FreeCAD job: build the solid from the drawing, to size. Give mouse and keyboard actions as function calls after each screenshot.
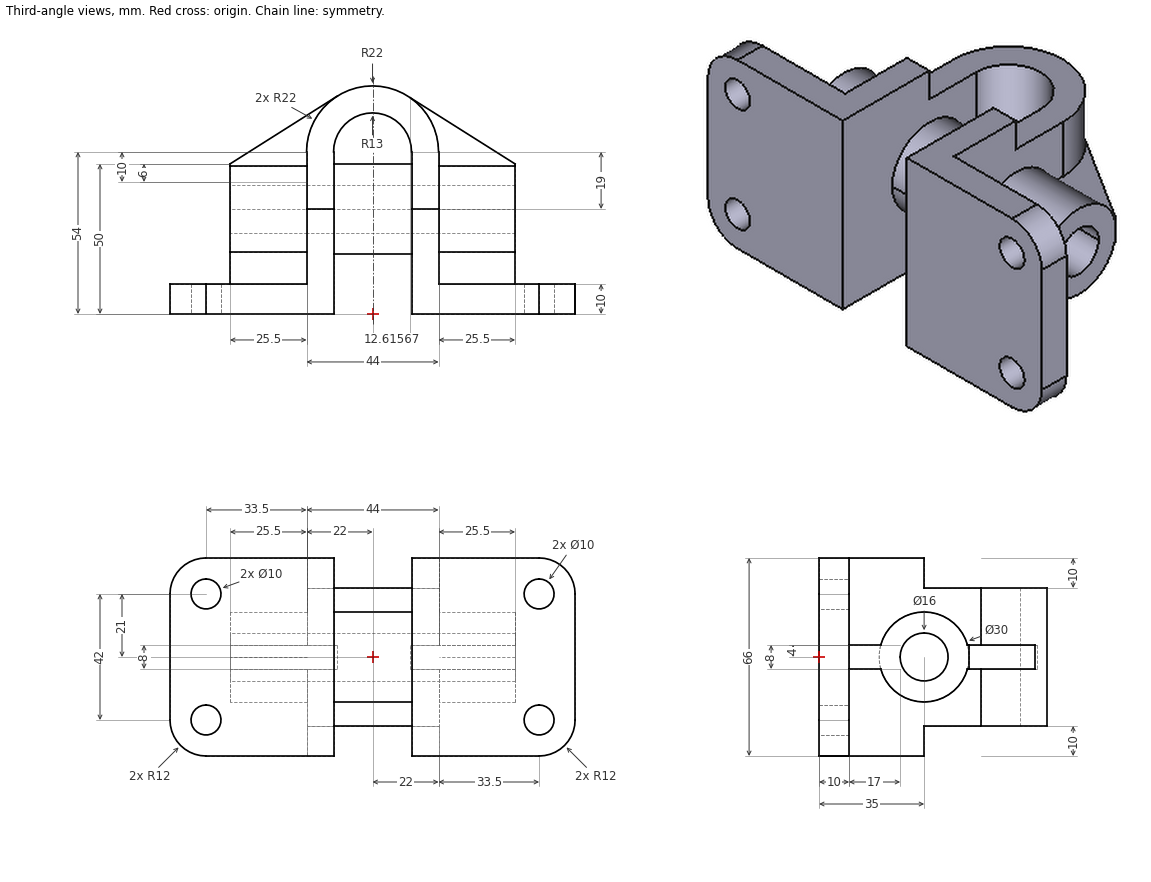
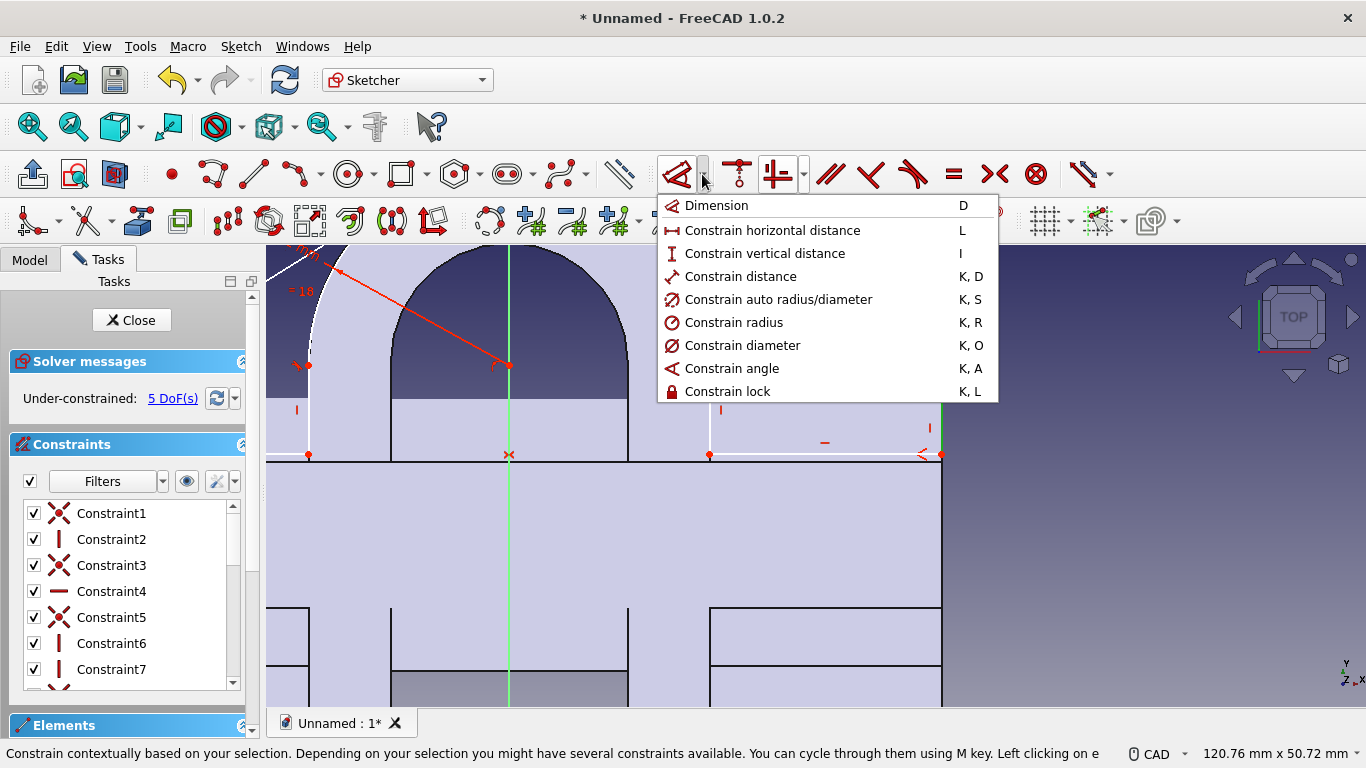
click(828, 254)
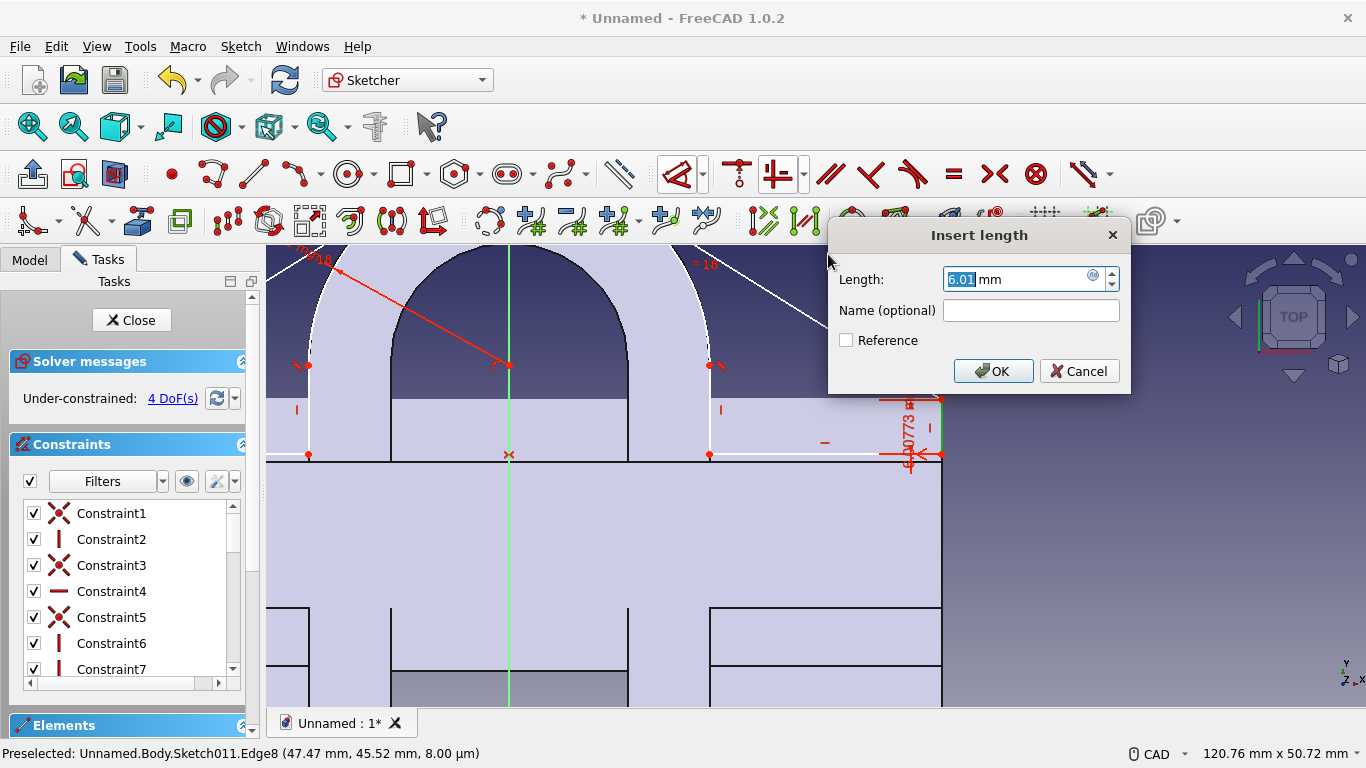
text(6)
key(Return)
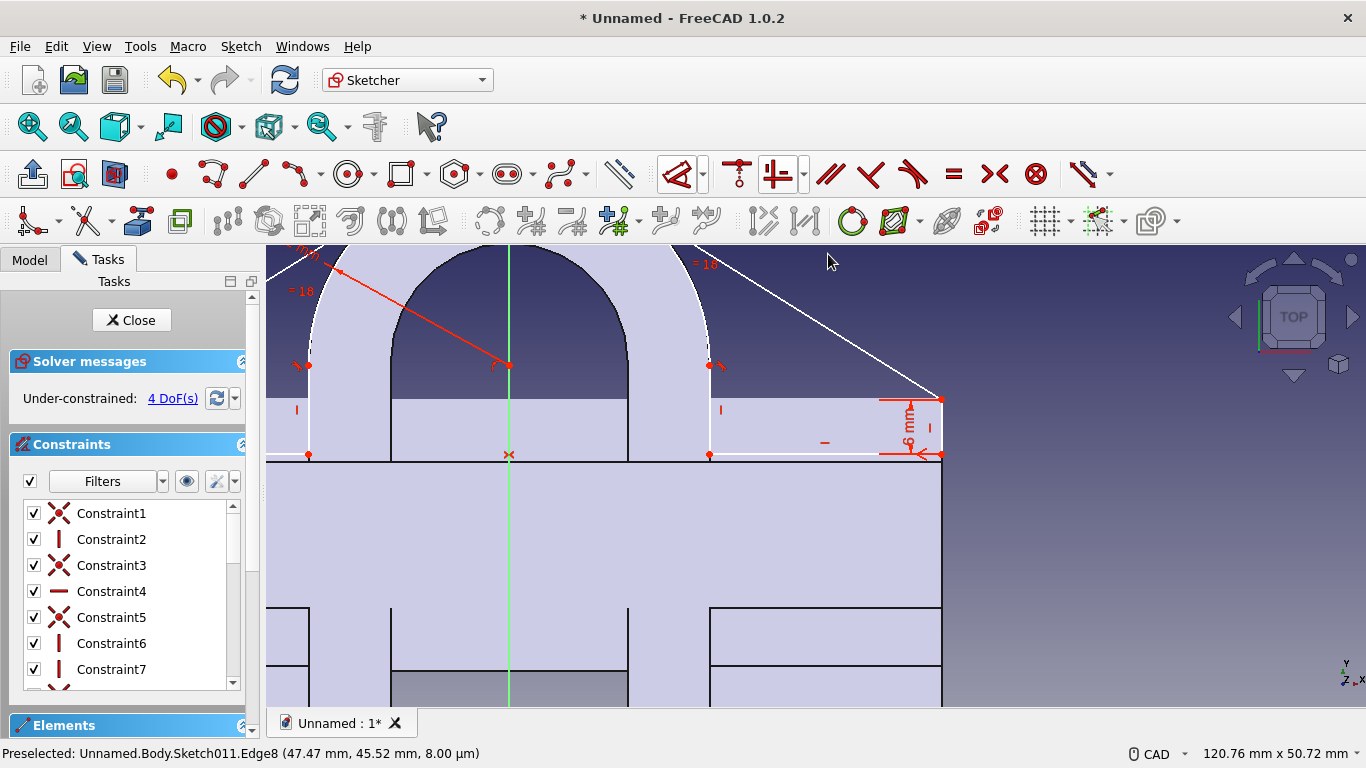
click(309, 428)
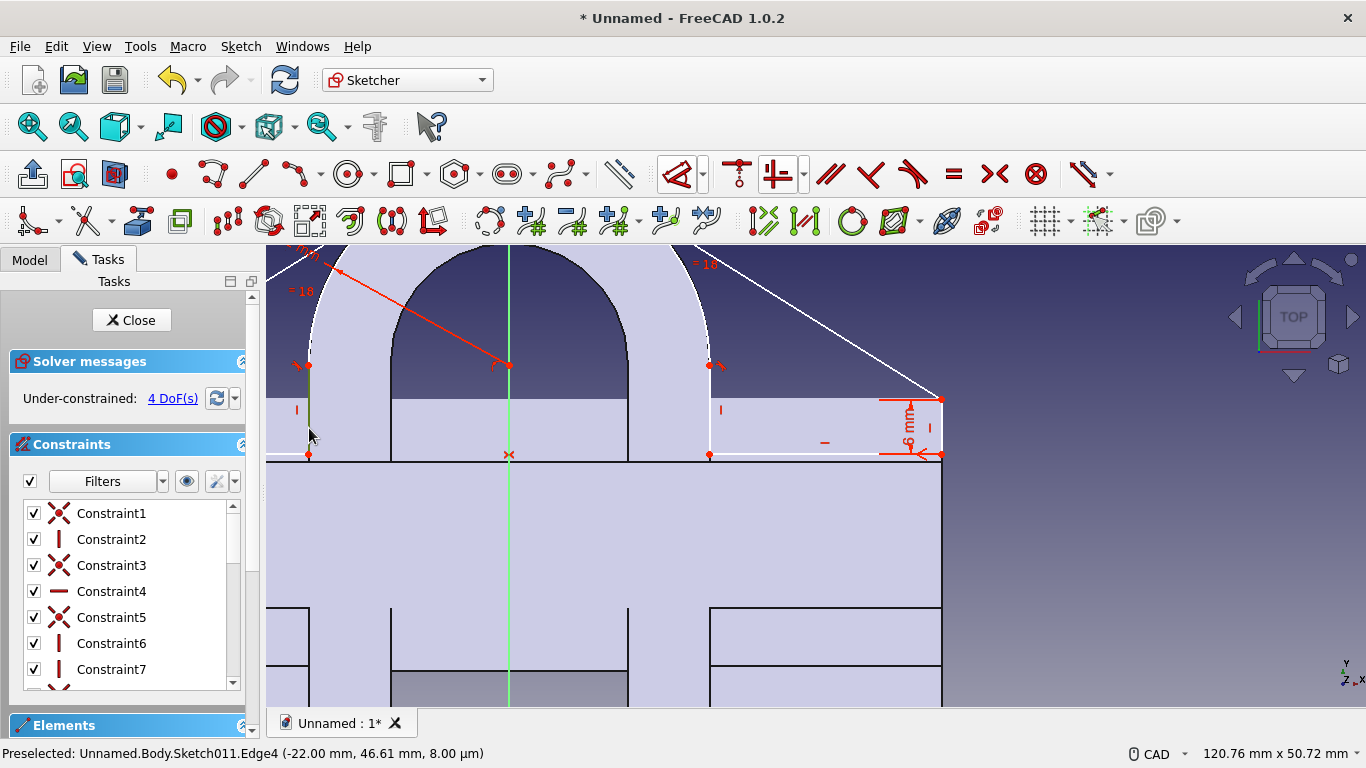
click(702, 174)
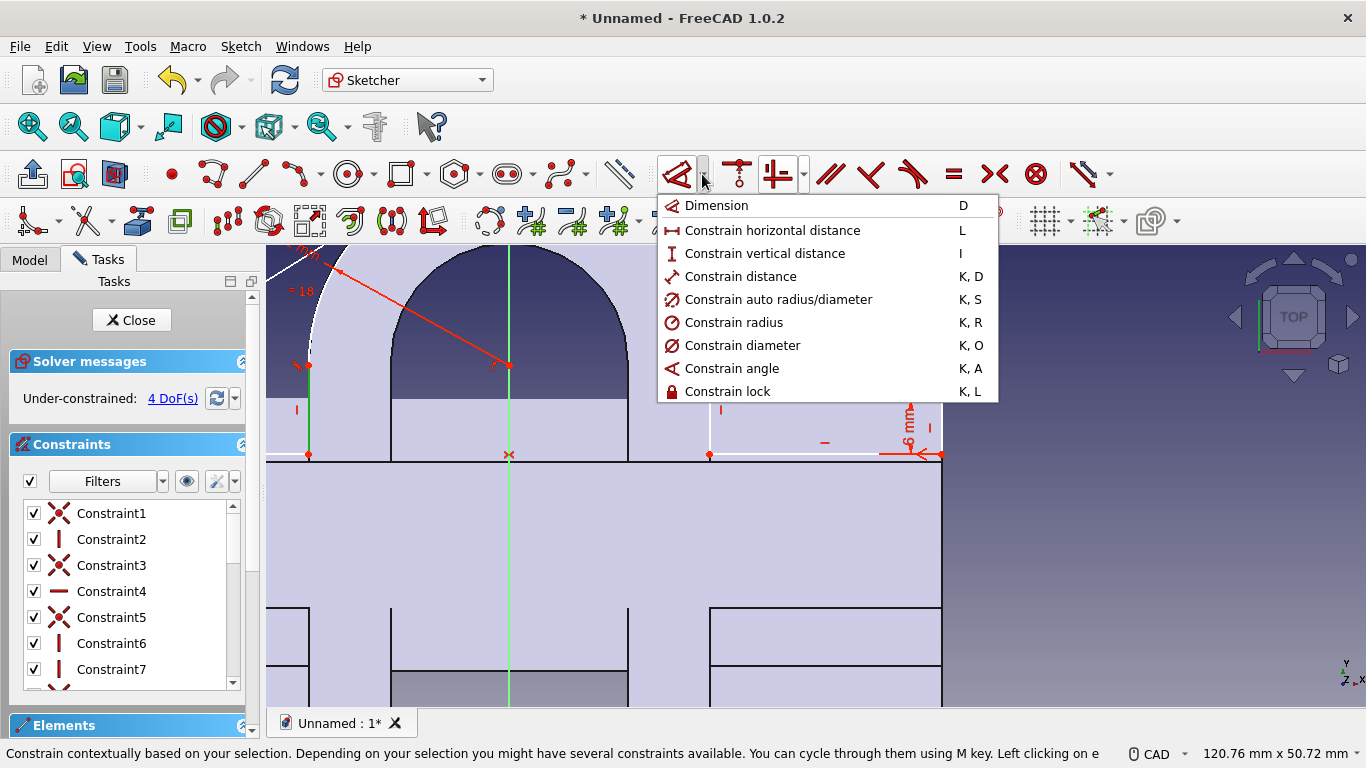
click(828, 254)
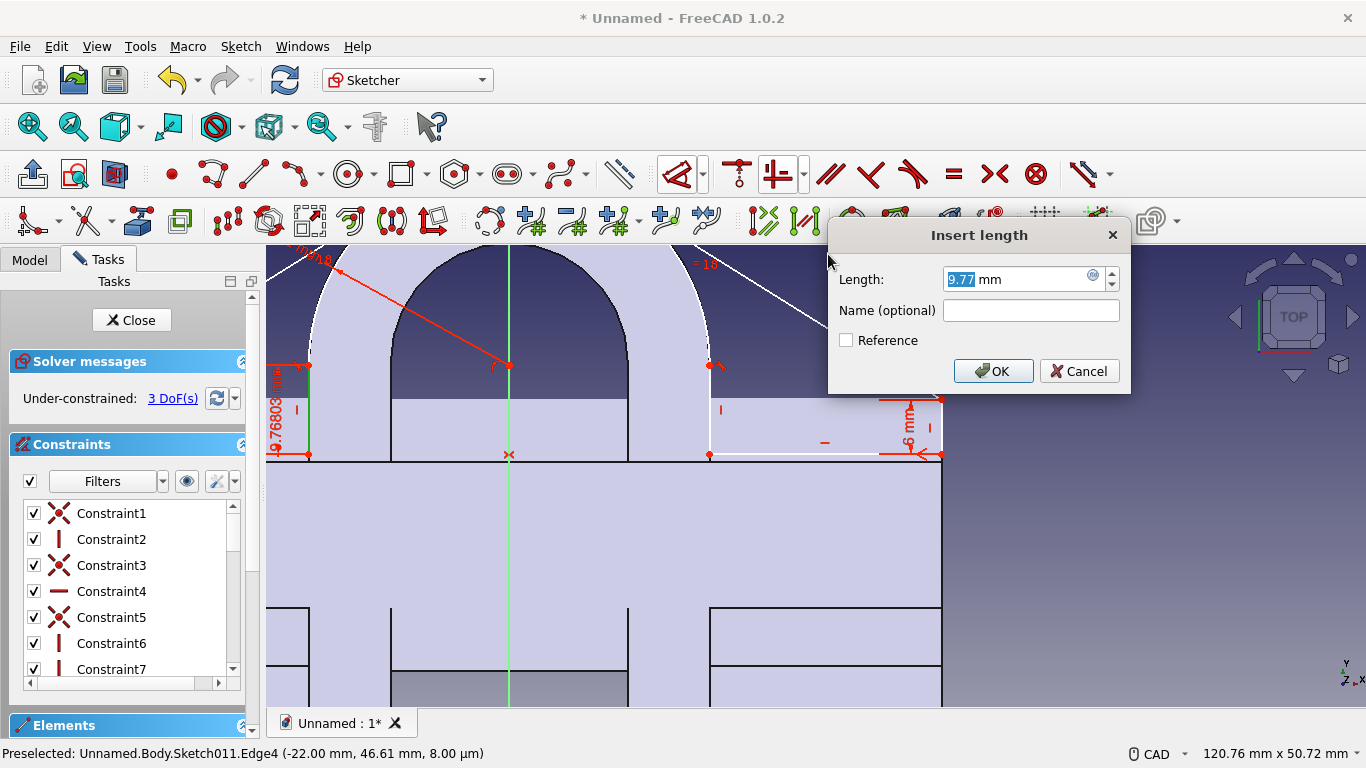
text(10)
key(Return)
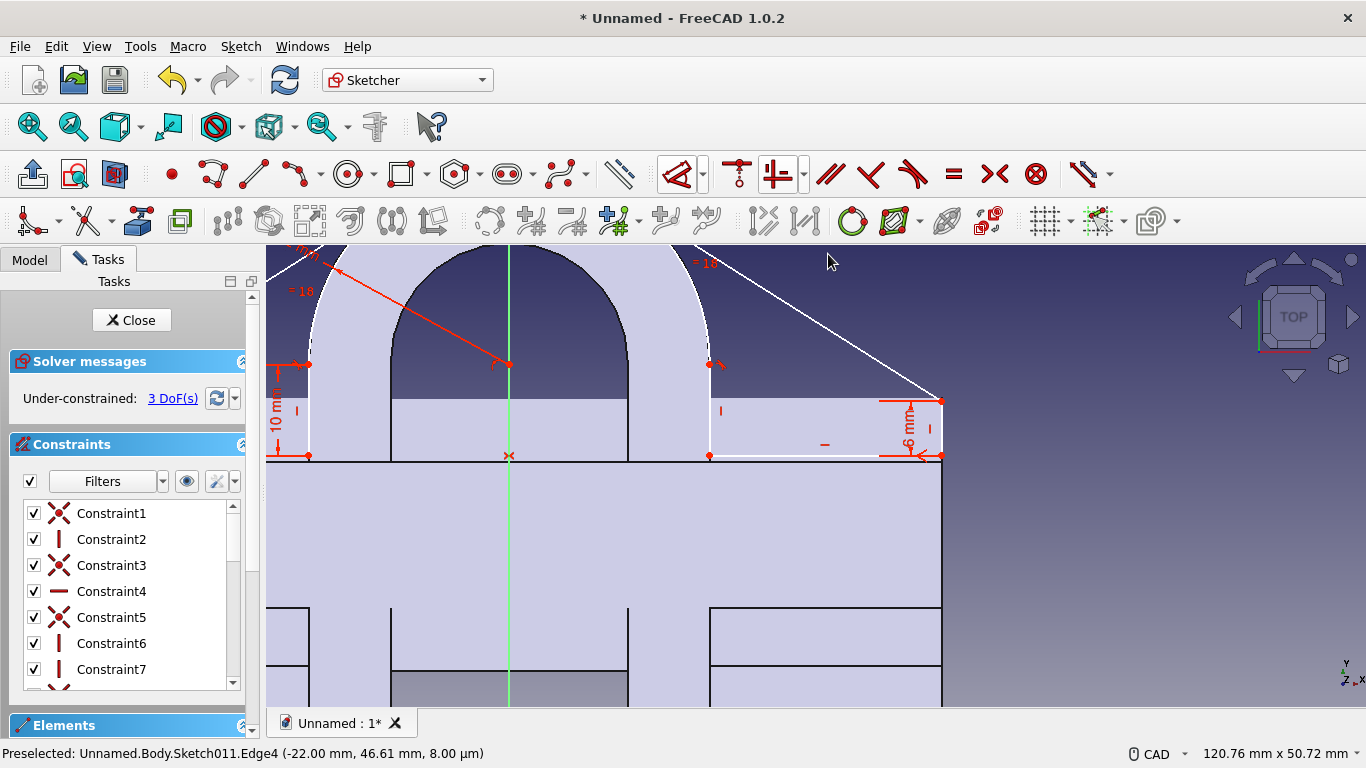
scroll(942, 438, down, 4)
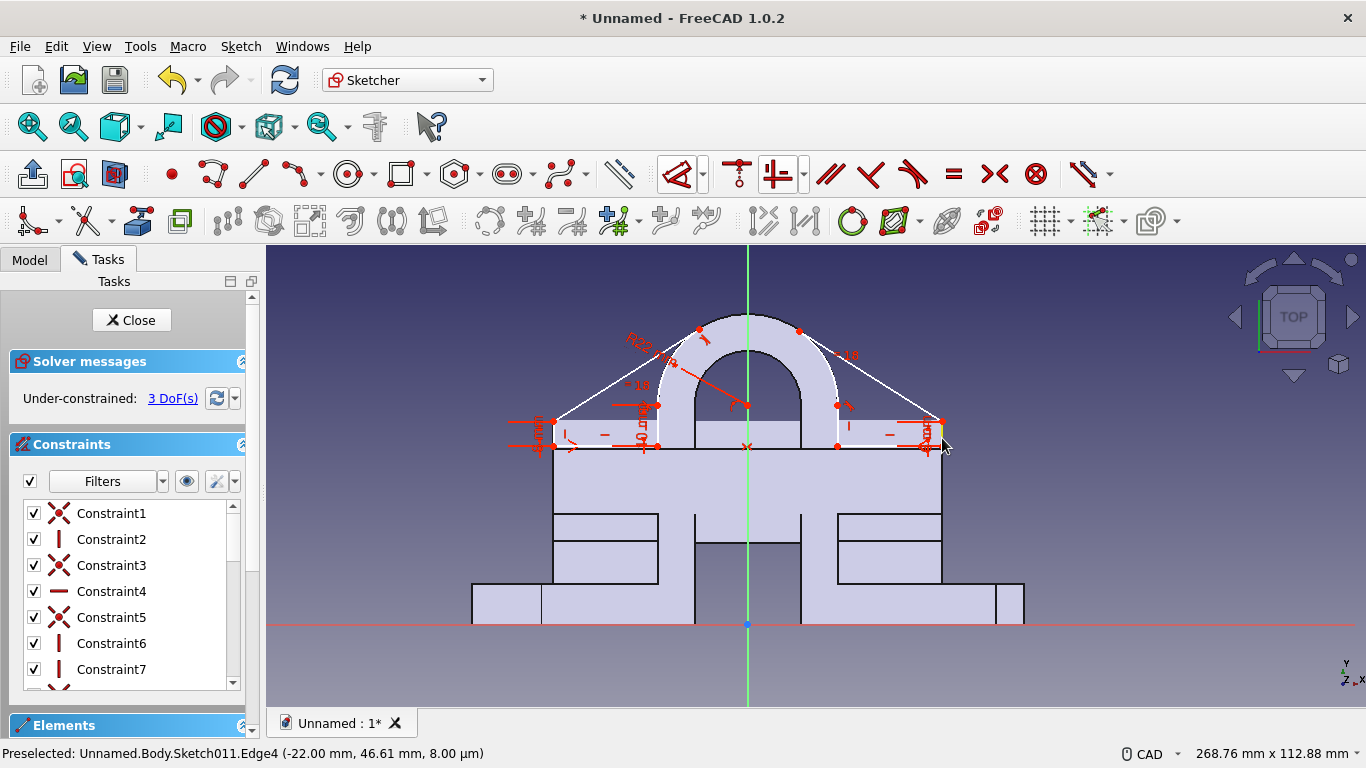
click(554, 422)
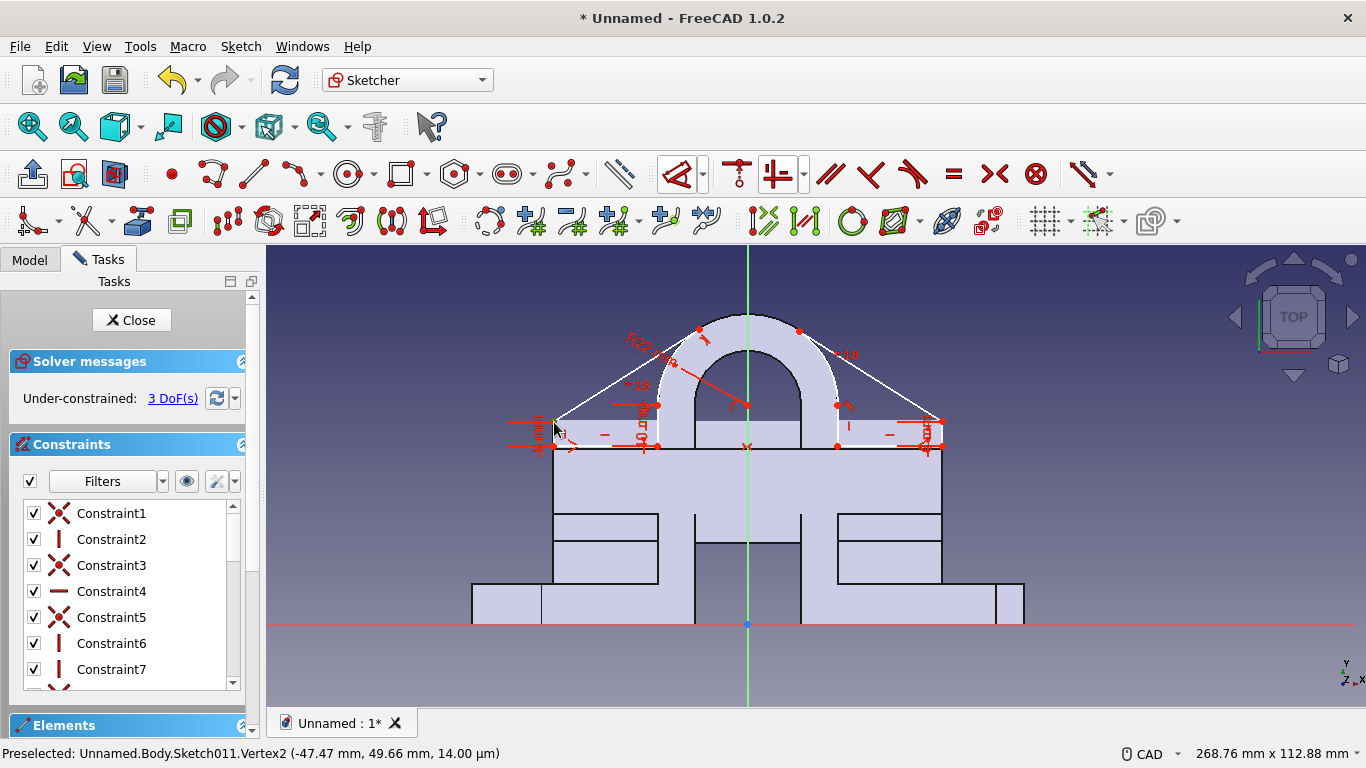
key(i)